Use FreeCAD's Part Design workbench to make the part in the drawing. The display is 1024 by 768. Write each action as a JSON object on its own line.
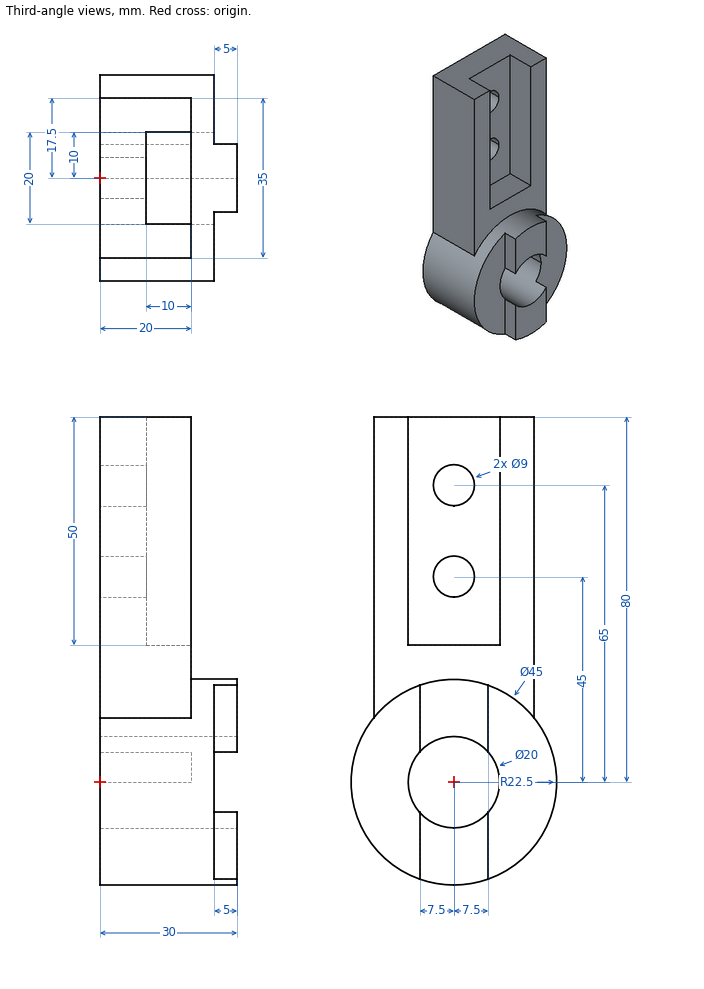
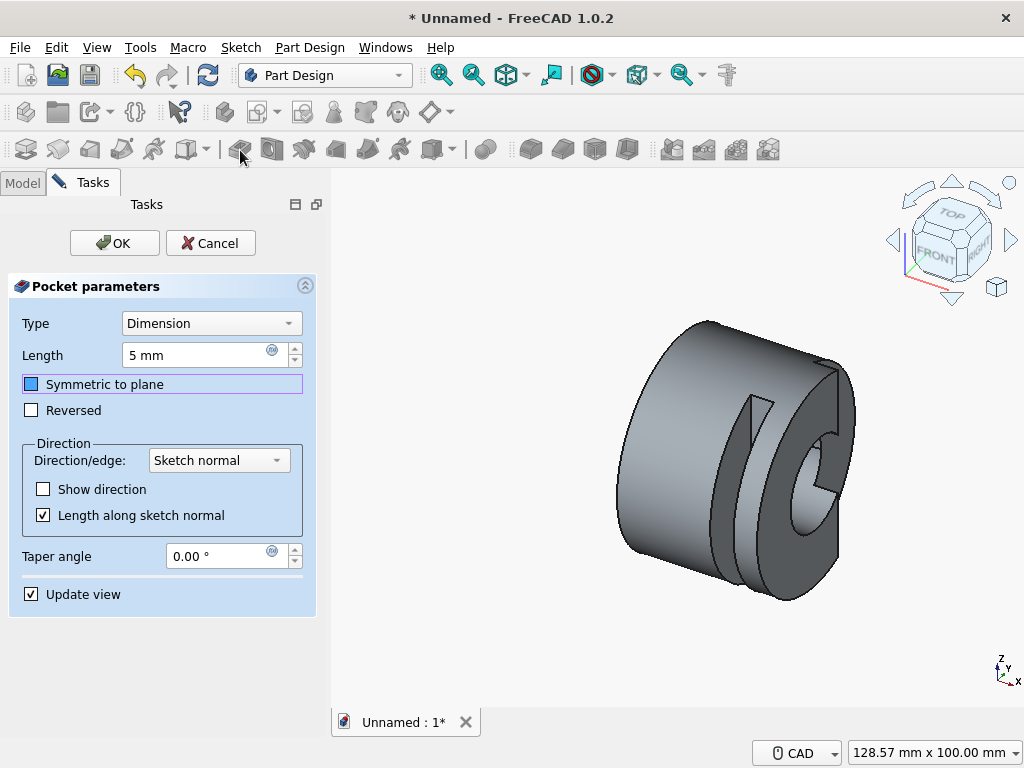
{"action": "left_click", "coordinate": [30, 410]}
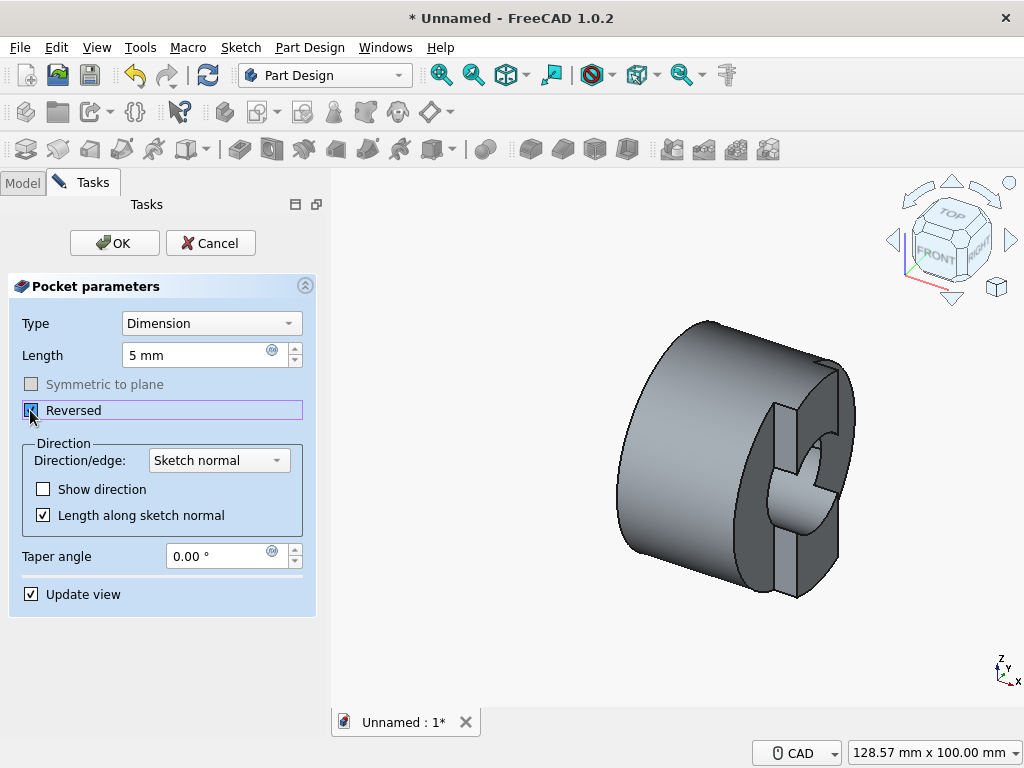
{"action": "left_click", "coordinate": [115, 243]}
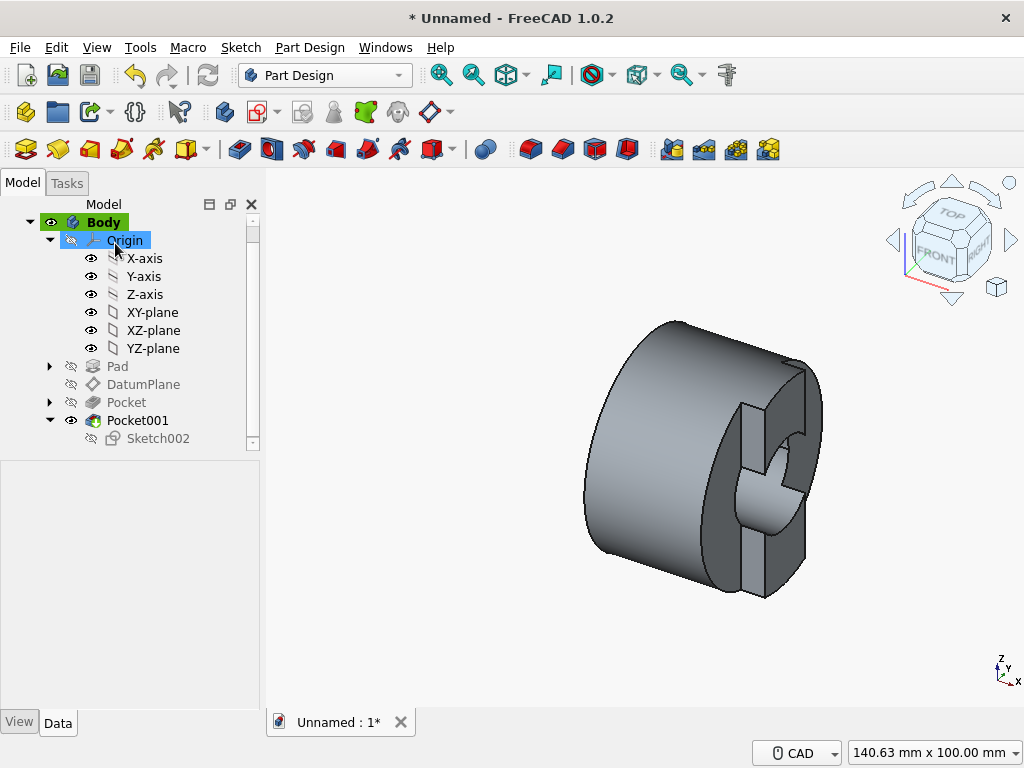
{"action": "left_click", "coordinate": [258, 112]}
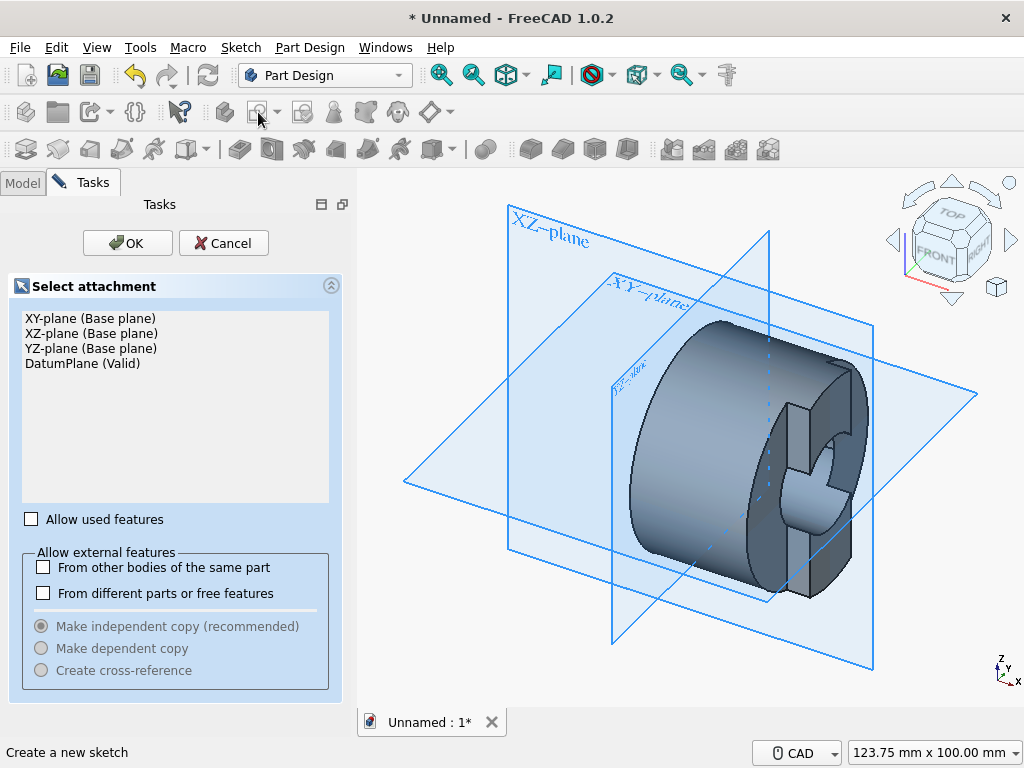
{"action": "left_click", "coordinate": [82, 318]}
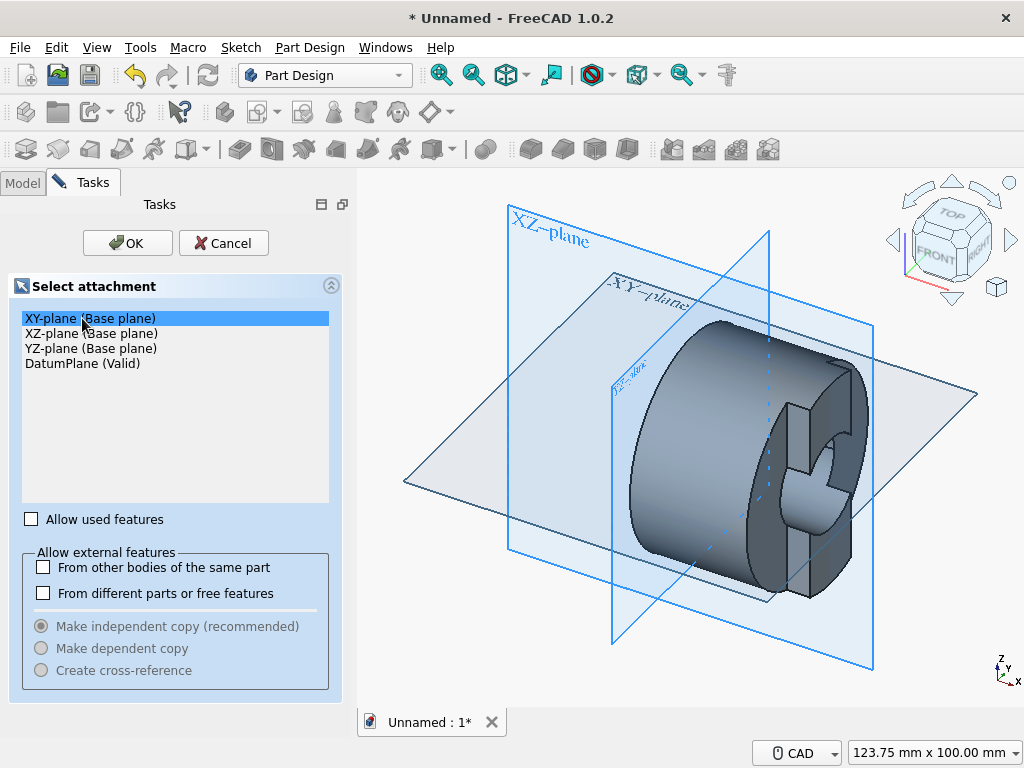
{"action": "left_click", "coordinate": [128, 243]}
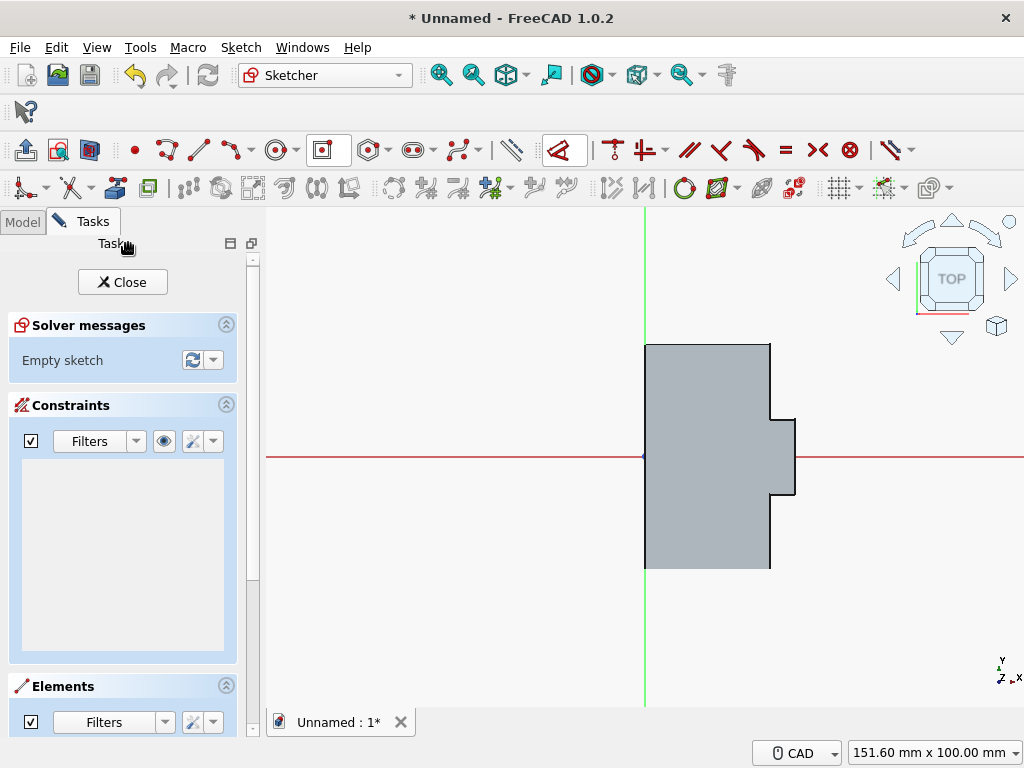
{"action": "left_click", "coordinate": [90, 150]}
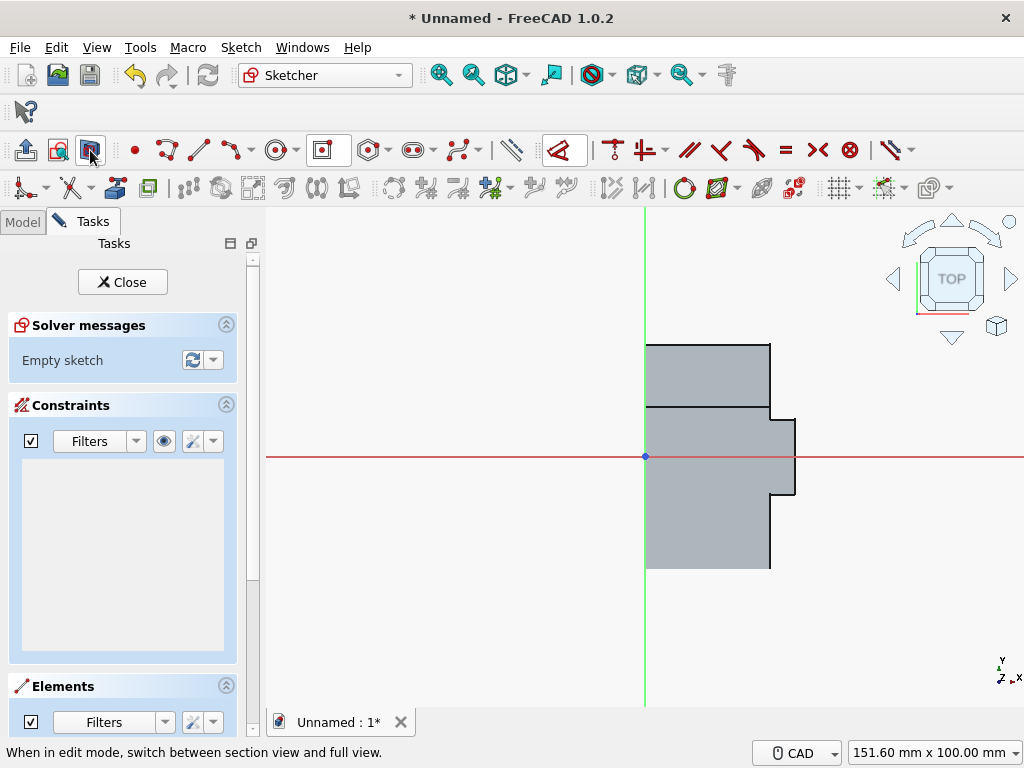
{"action": "scroll", "coordinate": [839, 457], "scroll_direction": "up", "scroll_amount": 3}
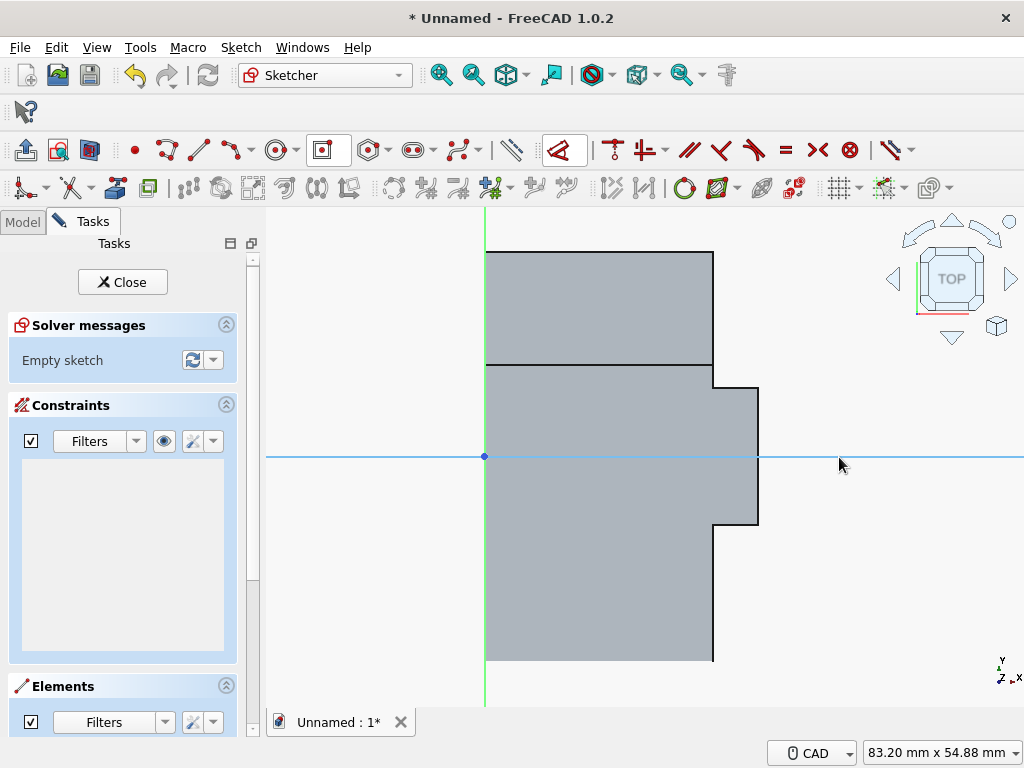
{"action": "left_click", "coordinate": [346, 150]}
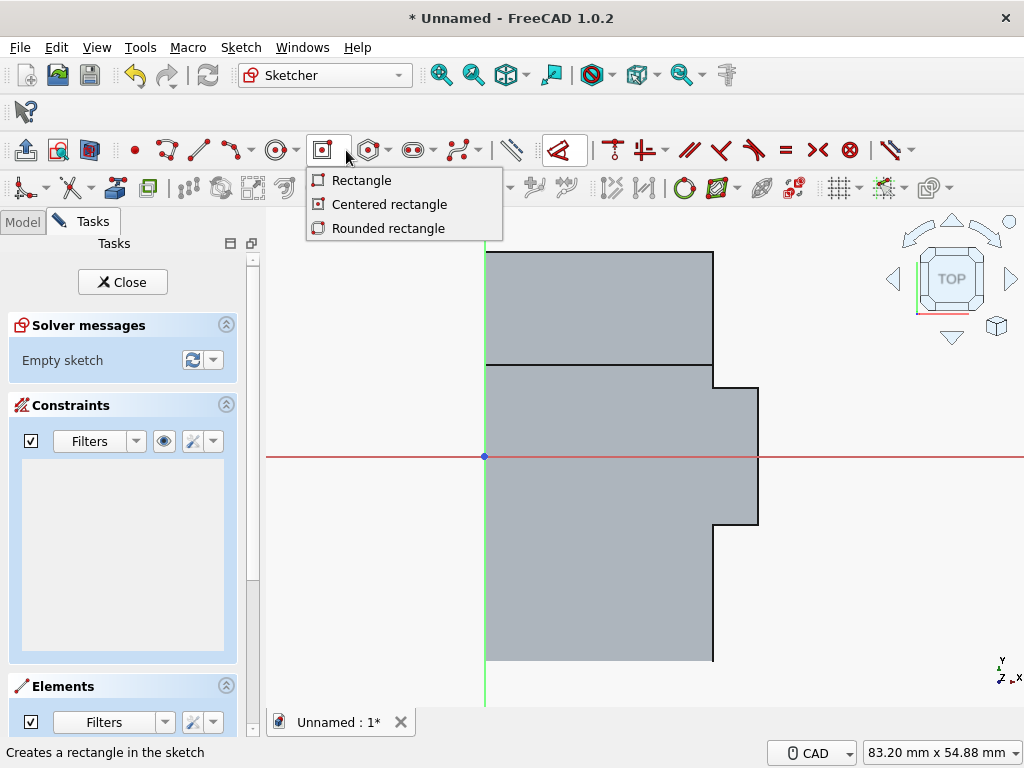
{"action": "left_click", "coordinate": [404, 180]}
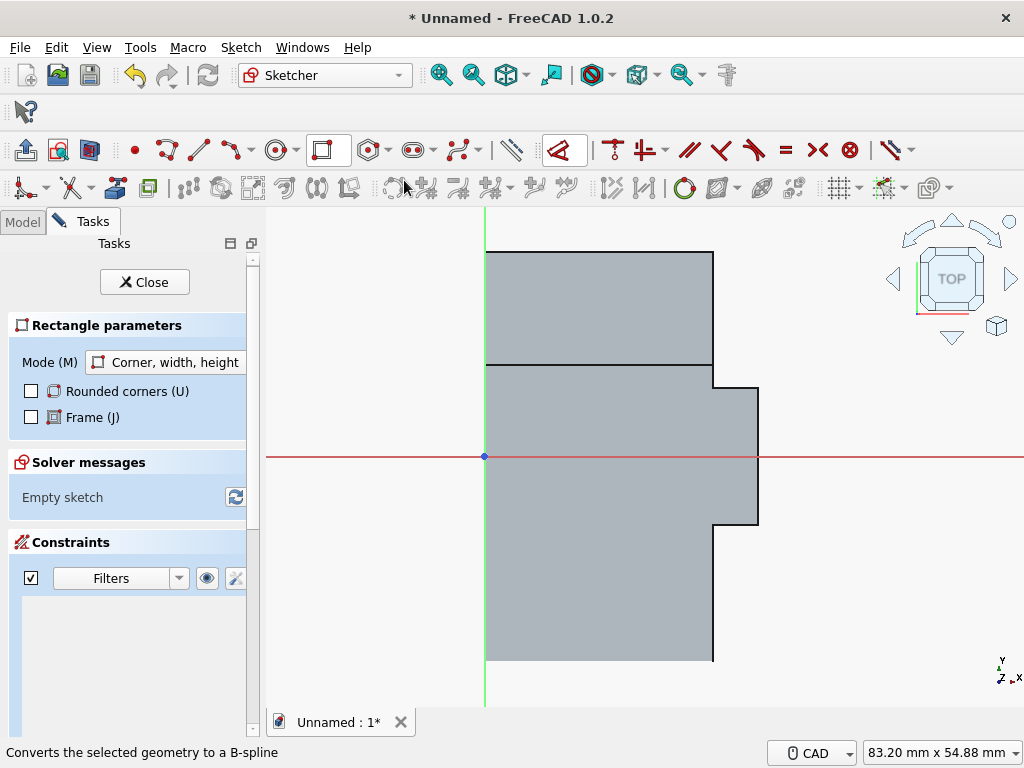
{"action": "left_click", "coordinate": [485, 297]}
{"action": "mouse_move", "coordinate": [667, 616]}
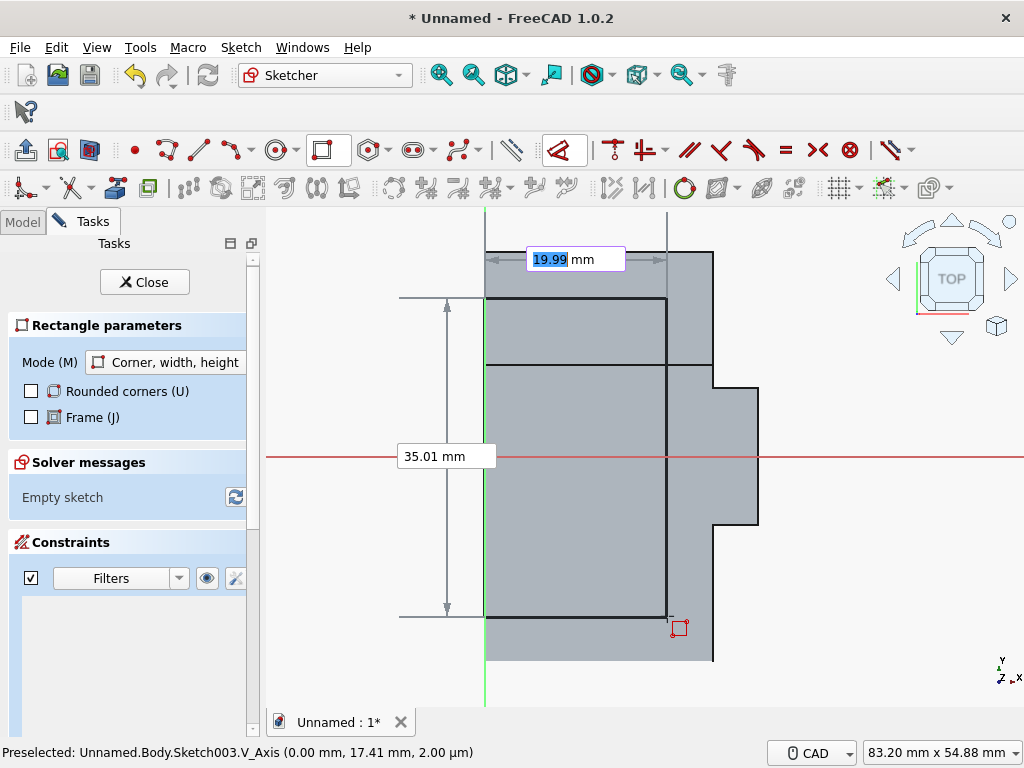
{"action": "type", "text": "20"}
{"action": "key", "text": "Tab"}
{"action": "type", "text": "35"}
{"action": "key", "text": "Return"}
{"action": "key", "text": "Escape"}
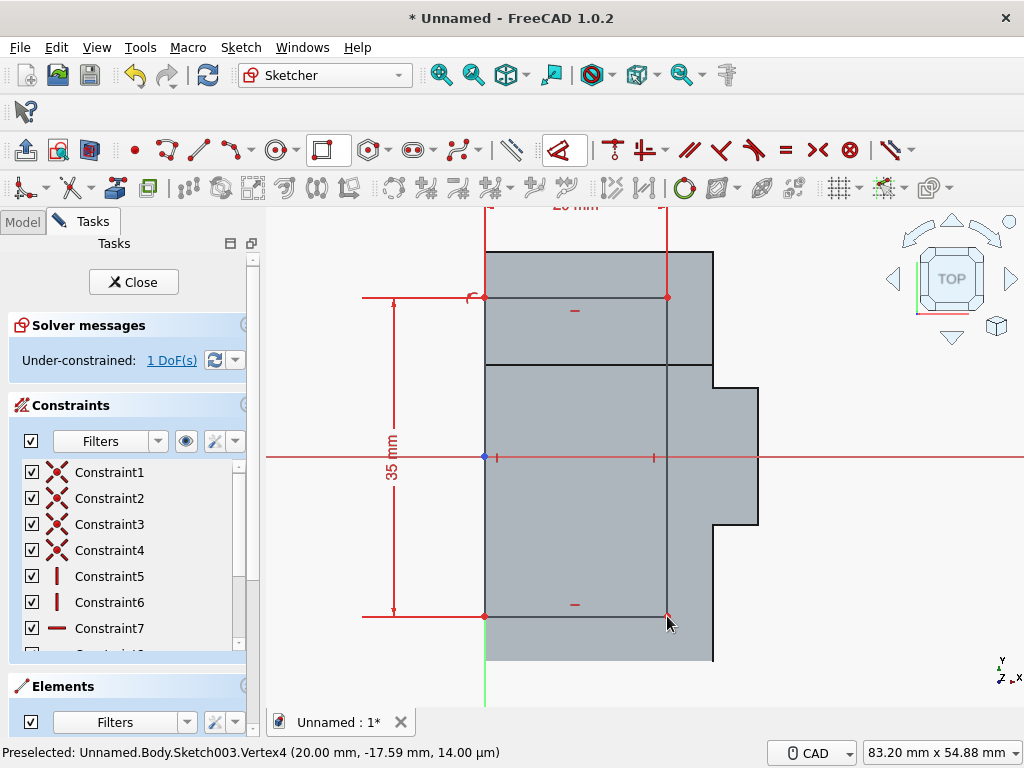
{"action": "left_click", "coordinate": [485, 298]}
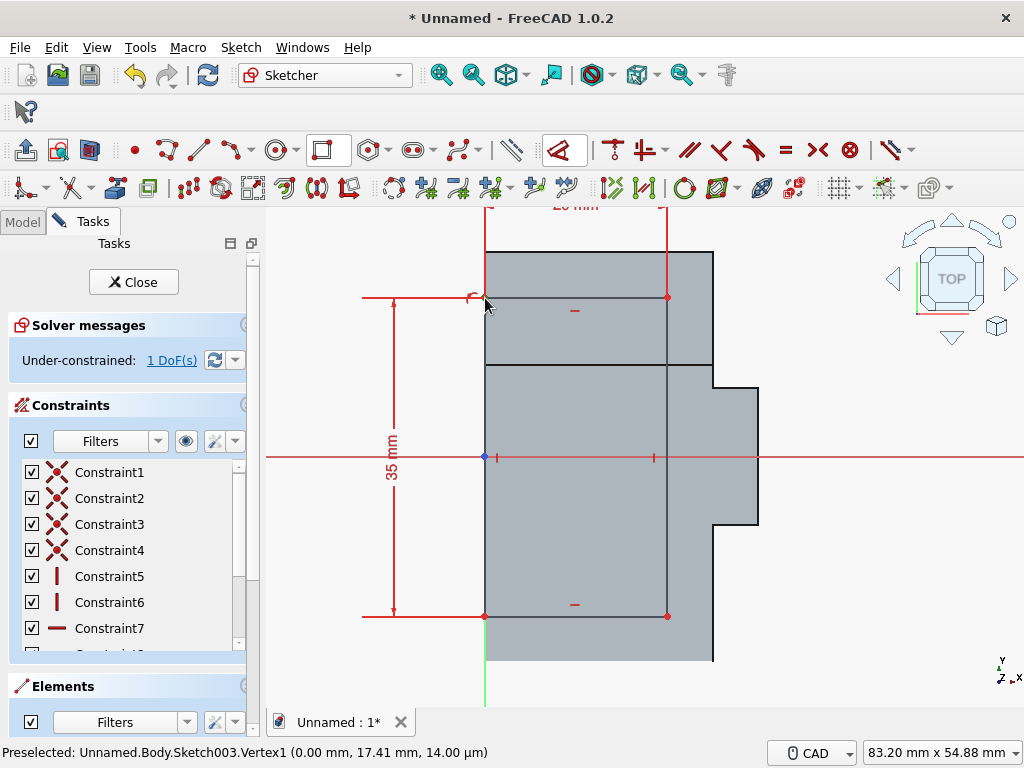
{"action": "key", "text": "i"}